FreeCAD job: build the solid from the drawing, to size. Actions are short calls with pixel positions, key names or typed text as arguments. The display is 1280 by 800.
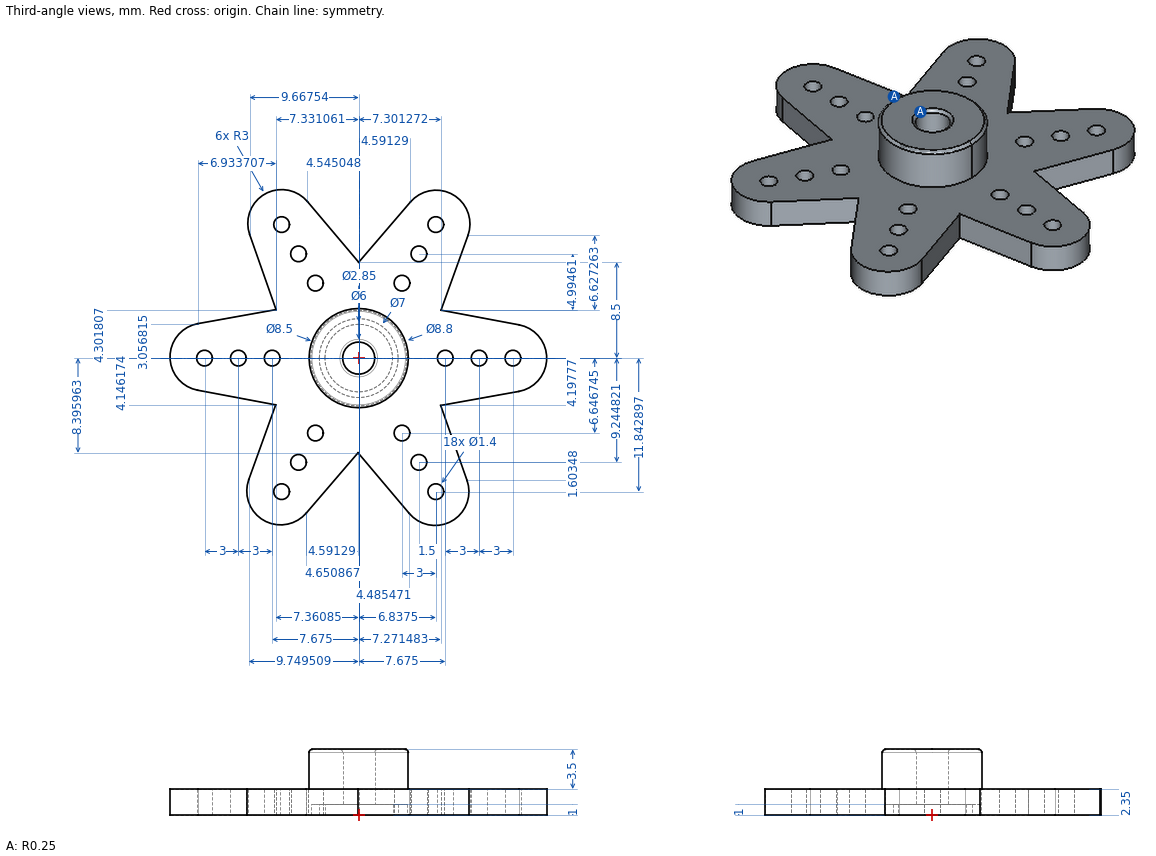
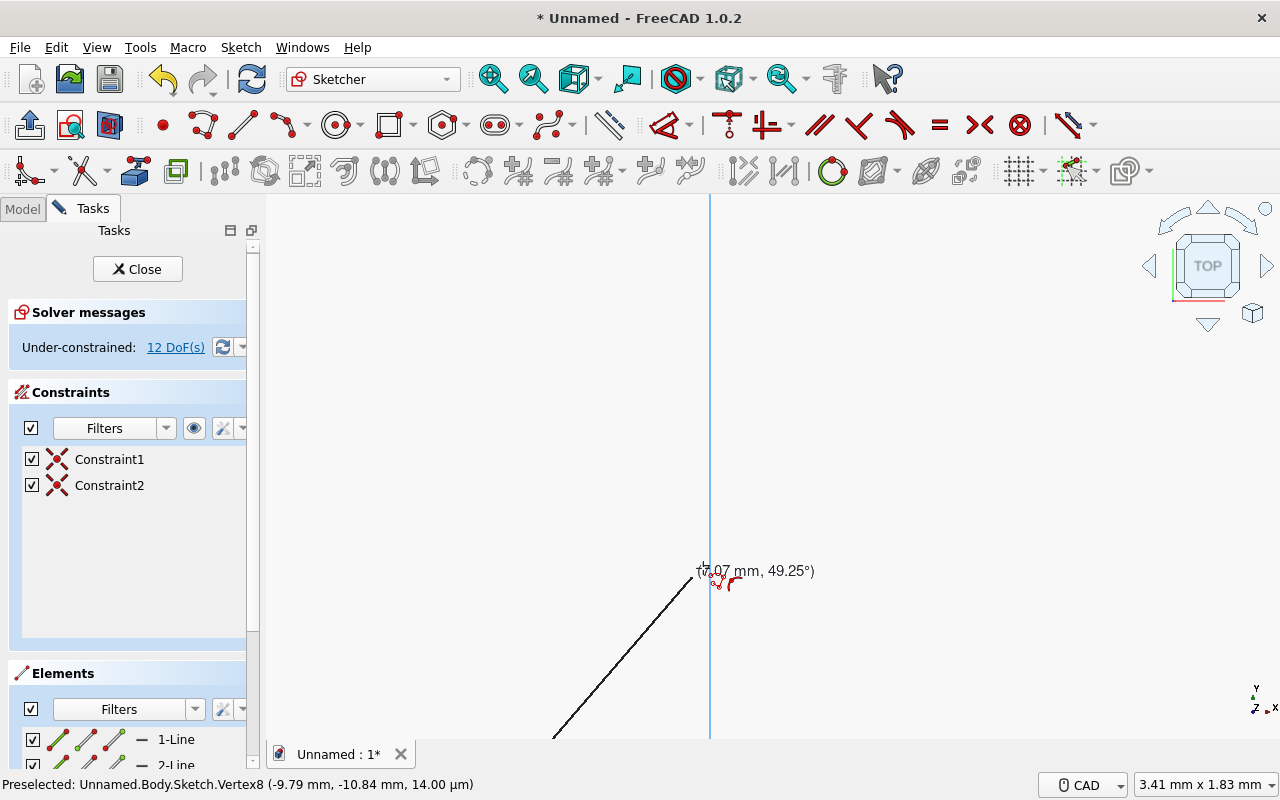
click(692, 560)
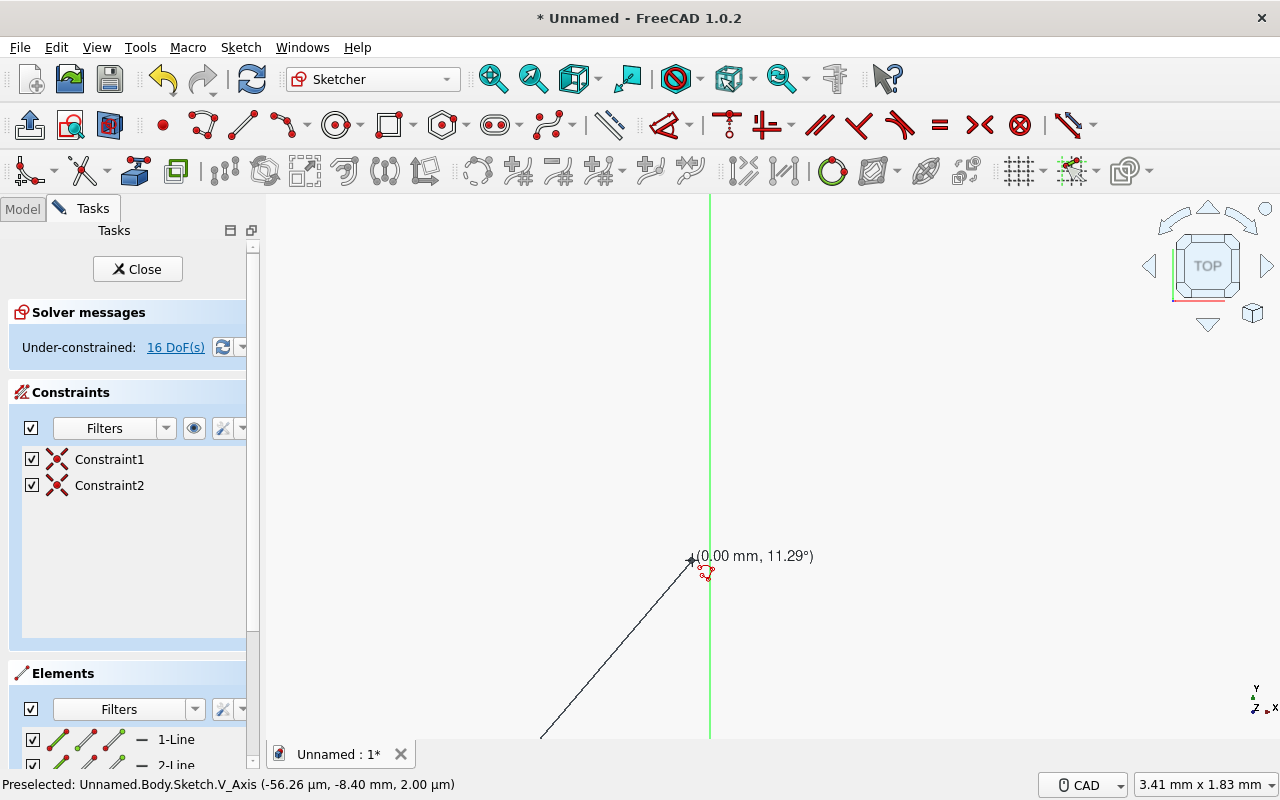
scroll(705, 593, down, 15)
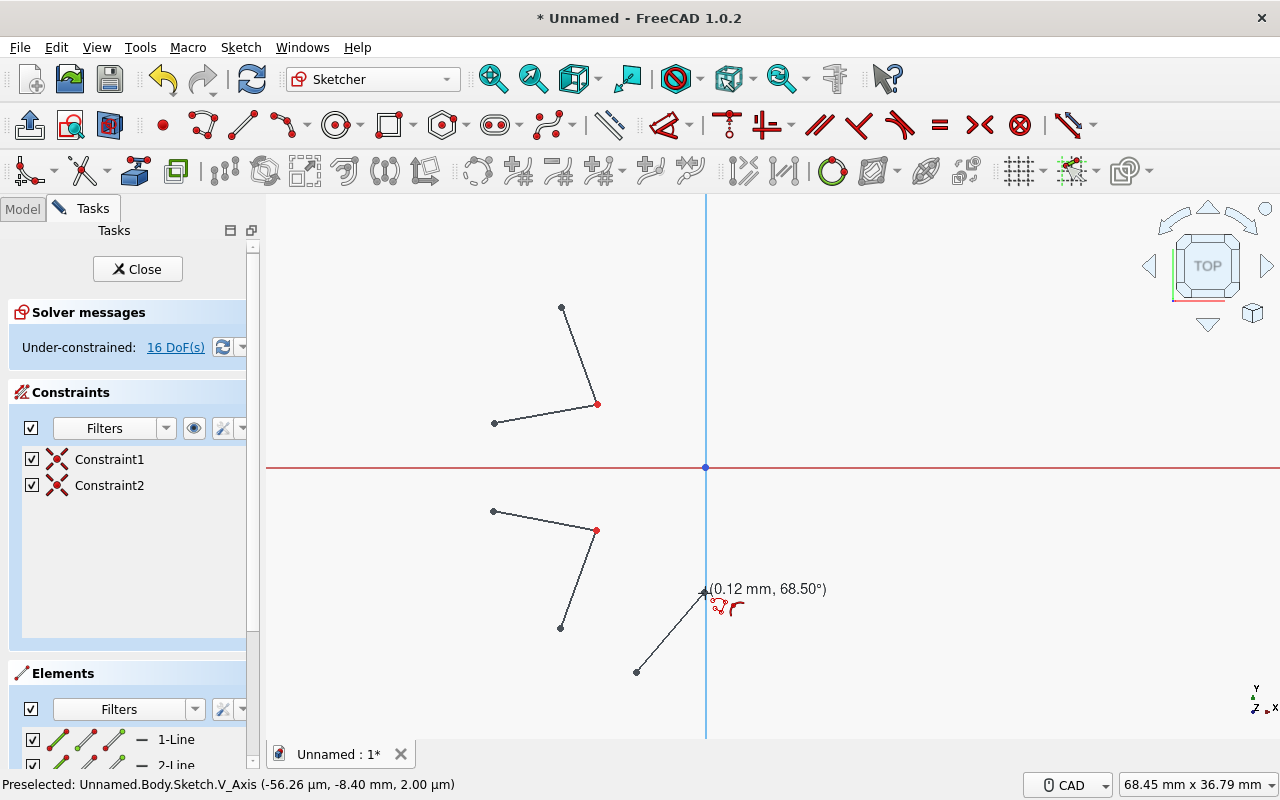
click(772, 672)
right_click(772, 672)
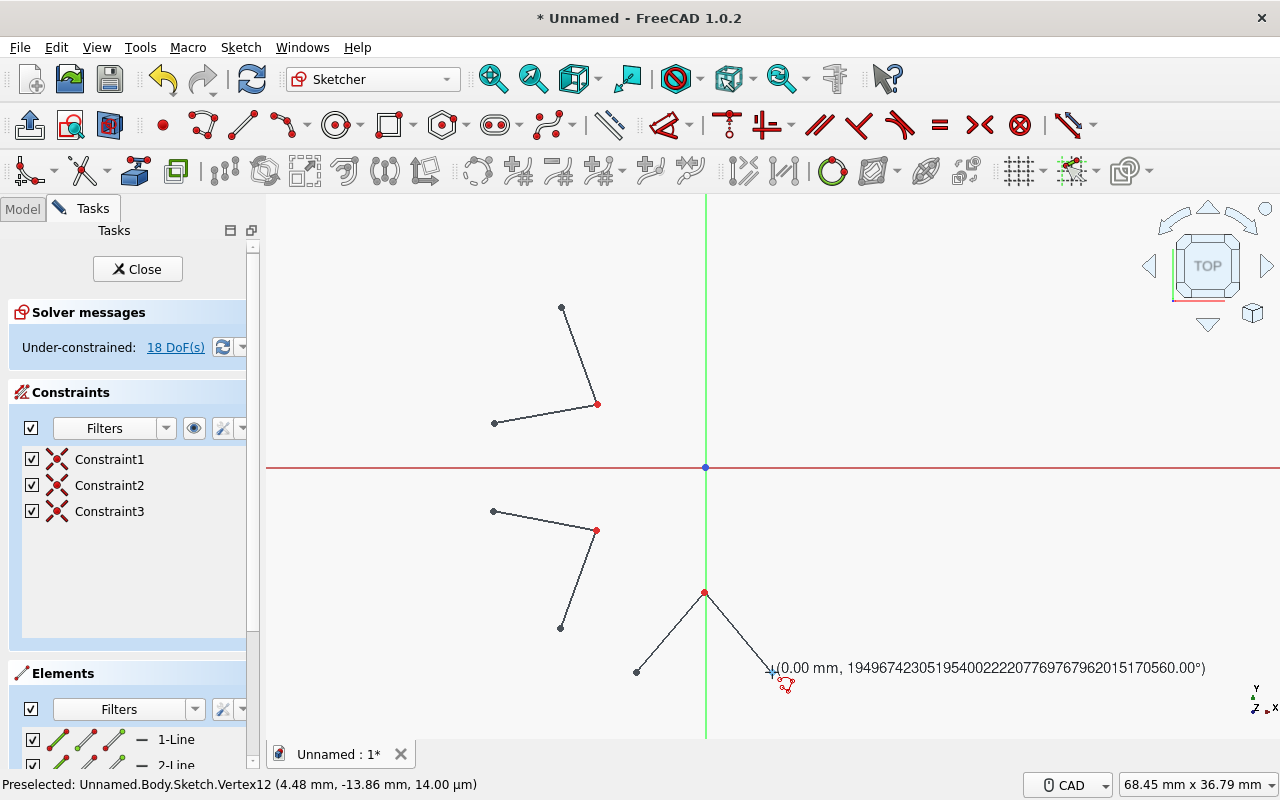
click(848, 628)
click(813, 530)
click(916, 511)
right_click(916, 511)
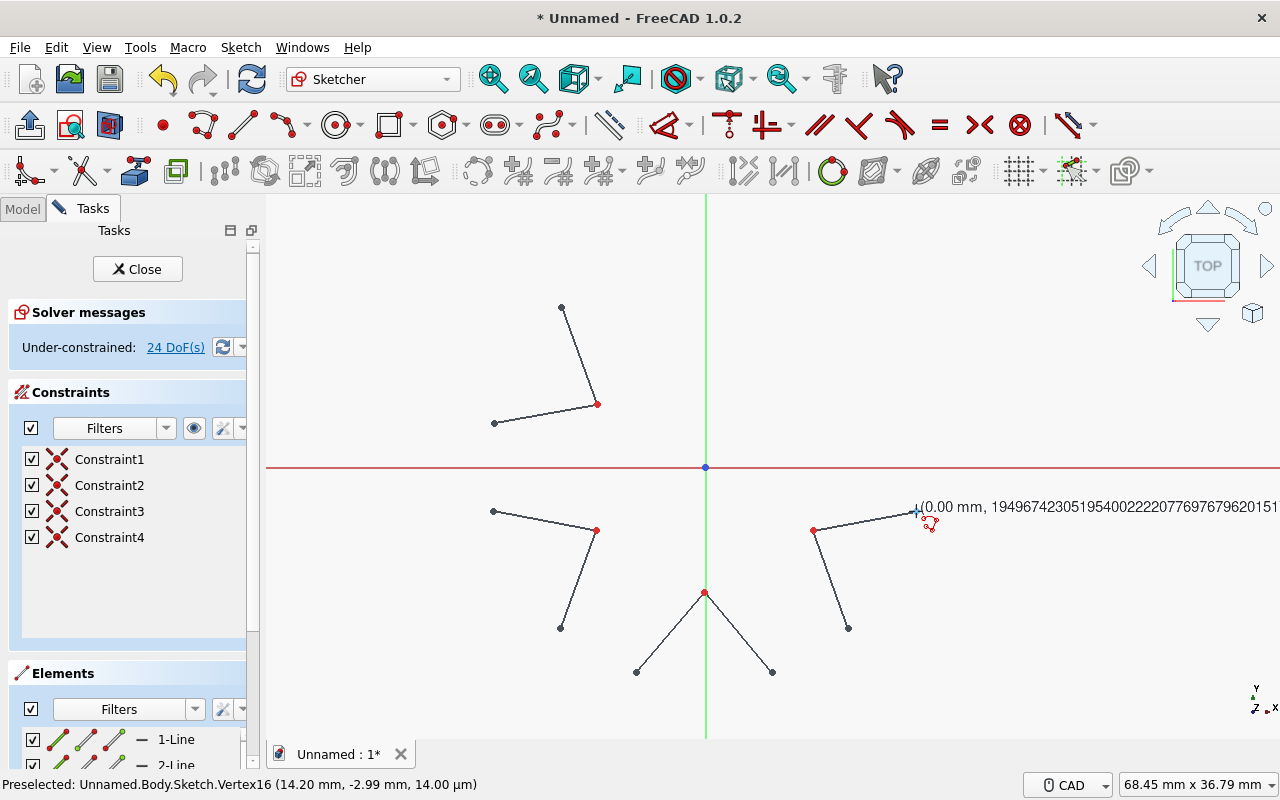
click(916, 424)
click(814, 405)
click(849, 307)
right_click(849, 307)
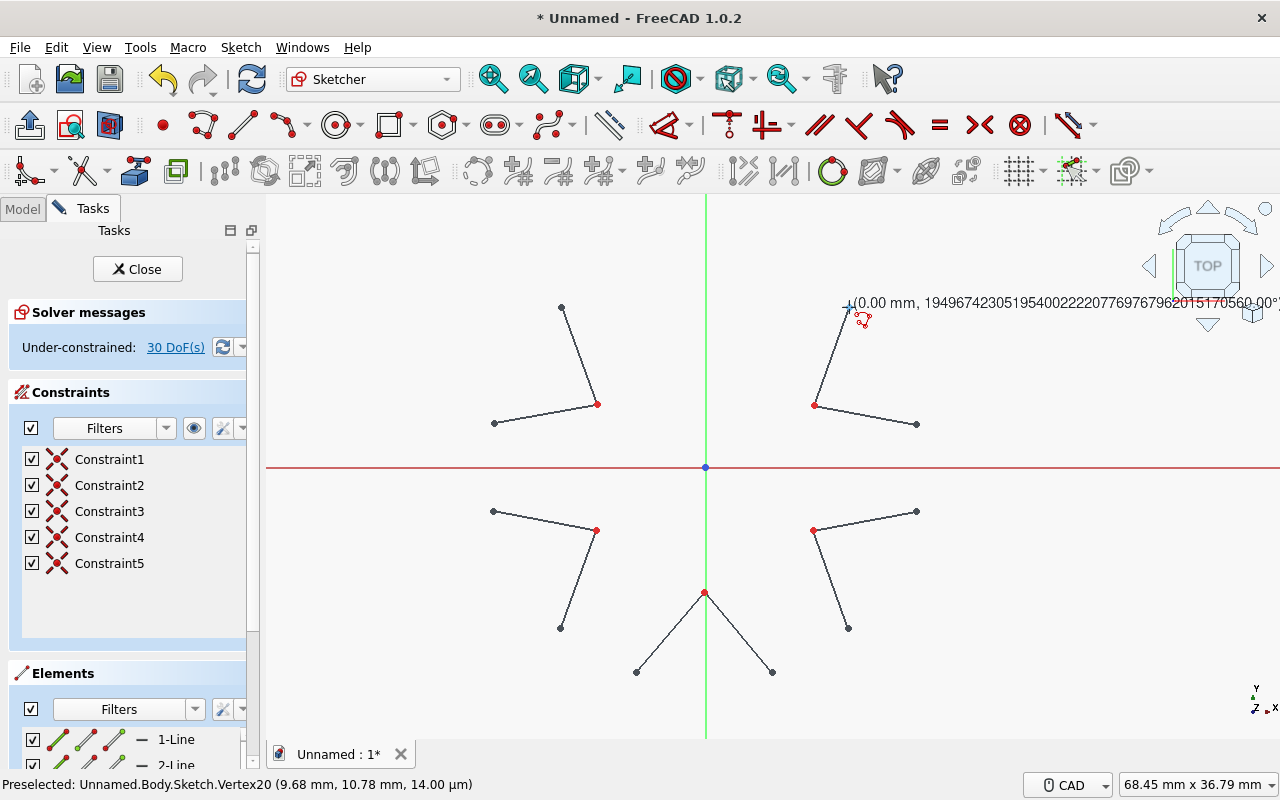
click(774, 263)
click(706, 342)
click(638, 262)
right_click(638, 262)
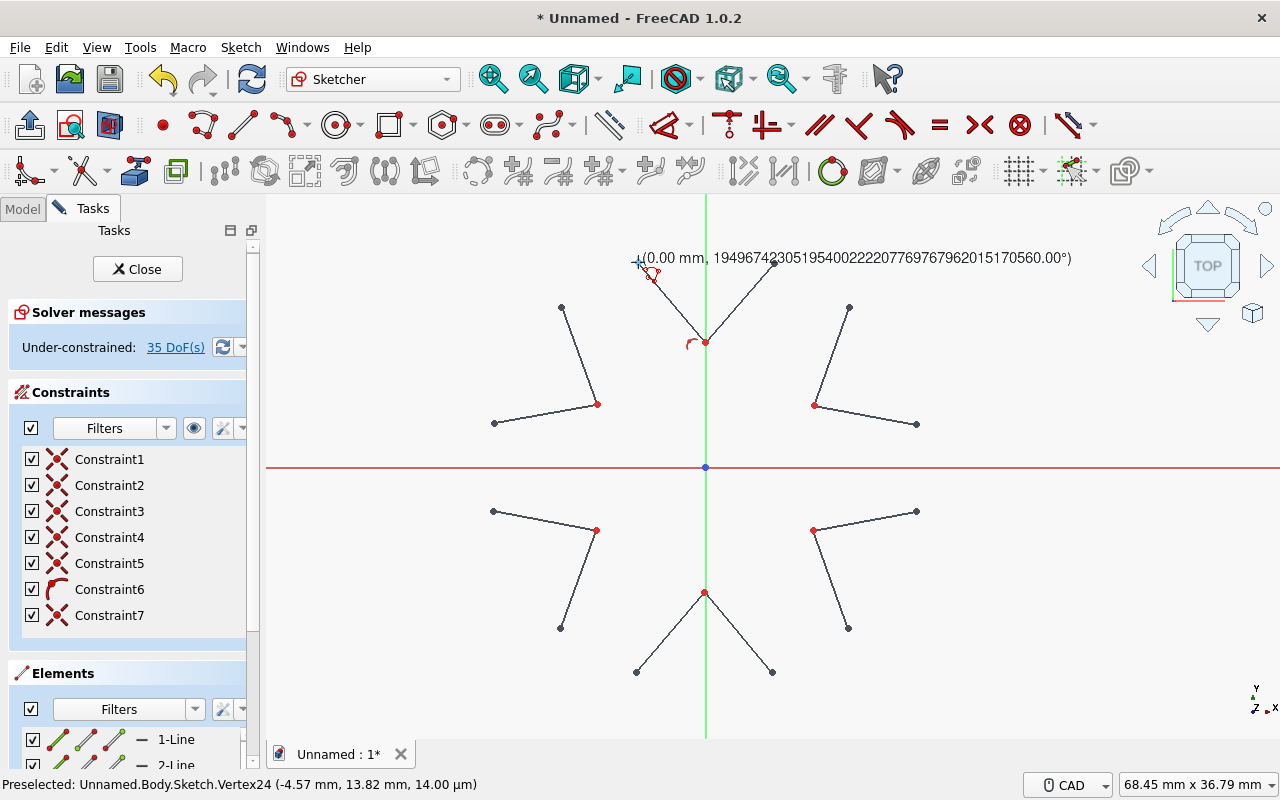
click(284, 126)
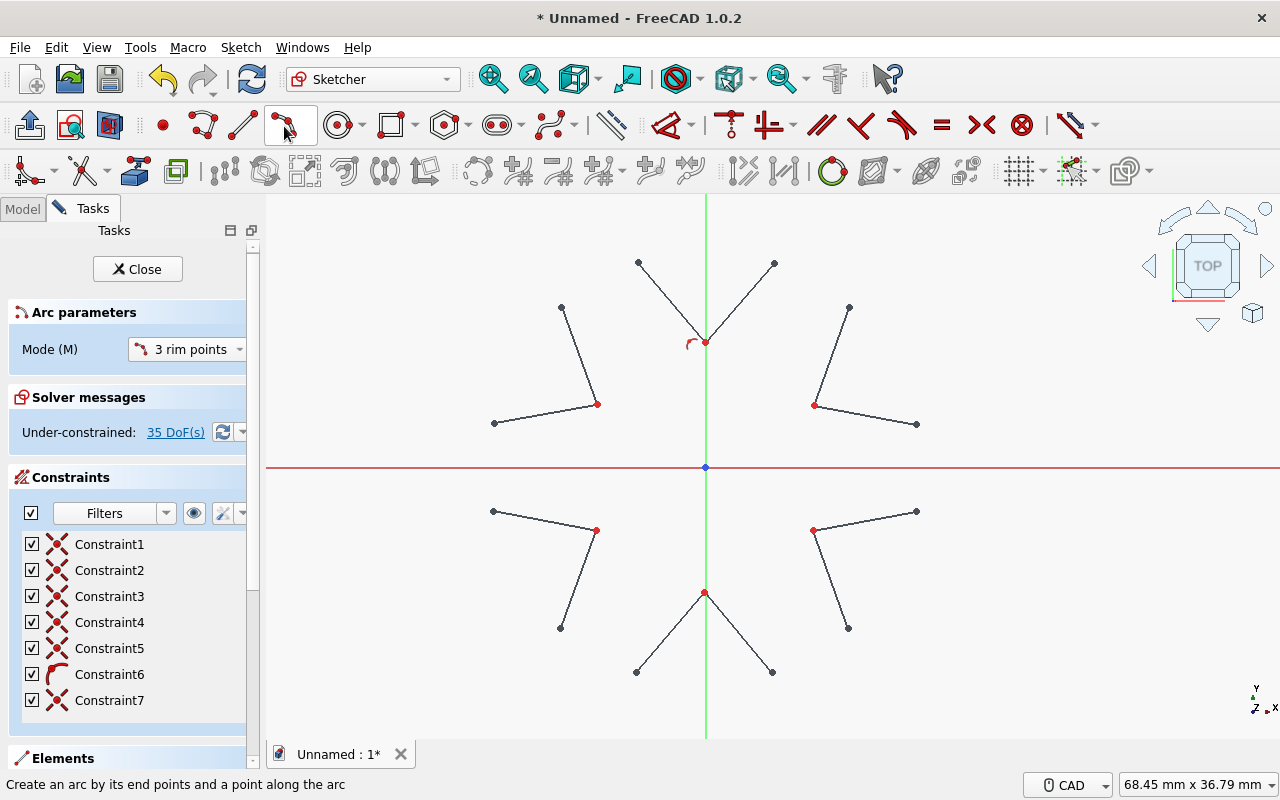
click(495, 423)
click(494, 511)
click(465, 443)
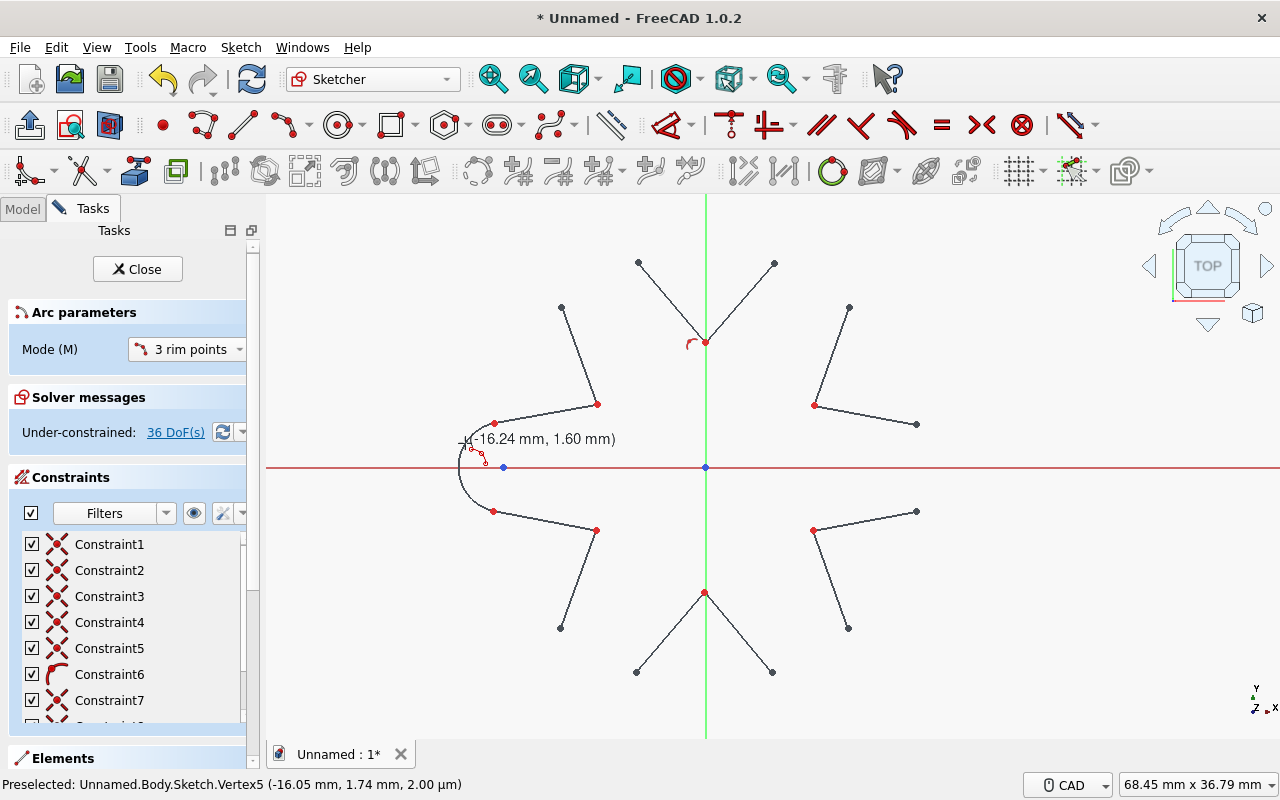
click(561, 628)
click(636, 672)
click(581, 681)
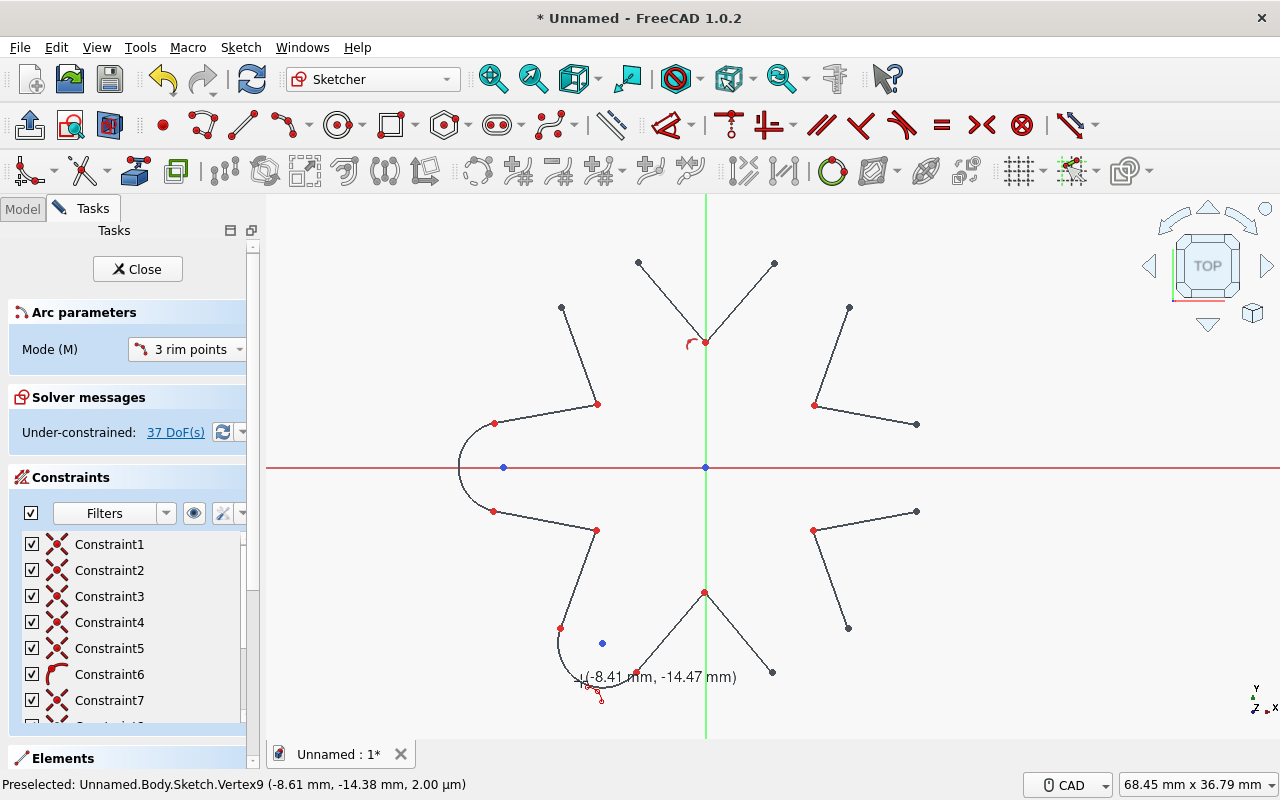
click(772, 673)
click(848, 629)
click(828, 682)